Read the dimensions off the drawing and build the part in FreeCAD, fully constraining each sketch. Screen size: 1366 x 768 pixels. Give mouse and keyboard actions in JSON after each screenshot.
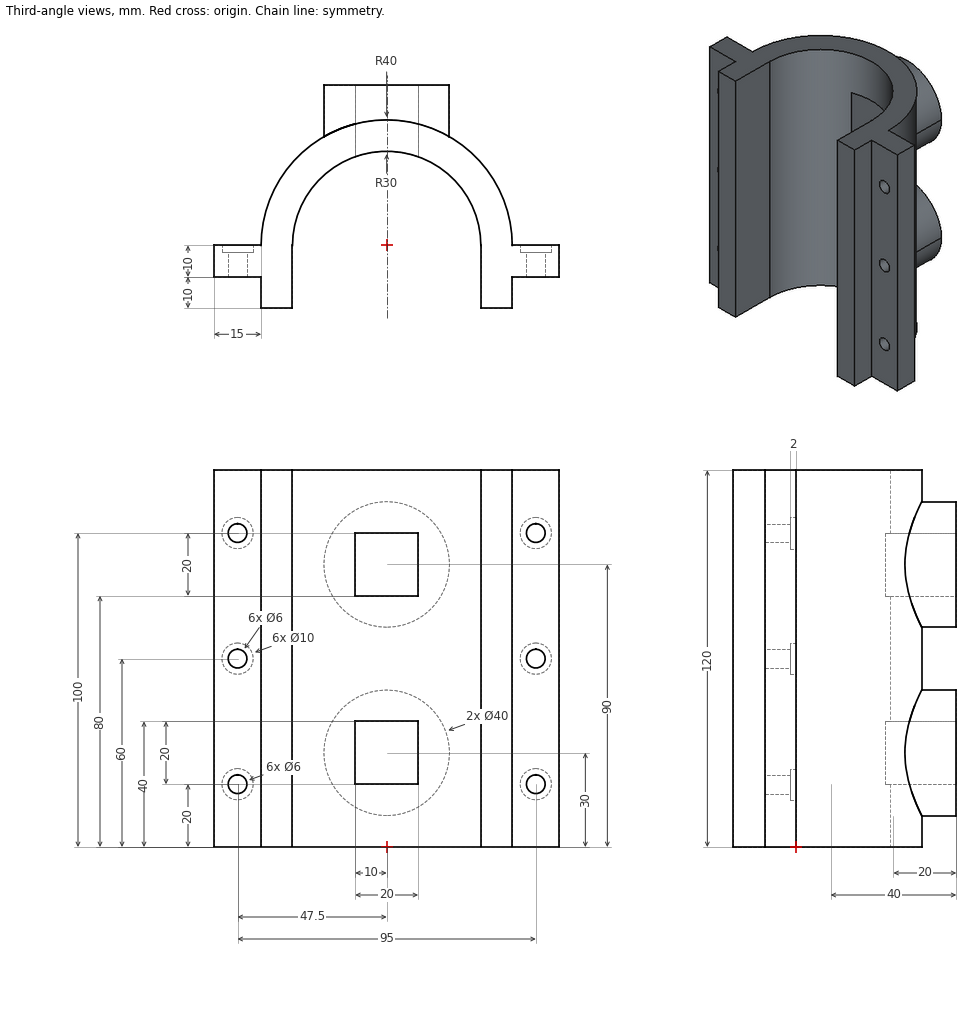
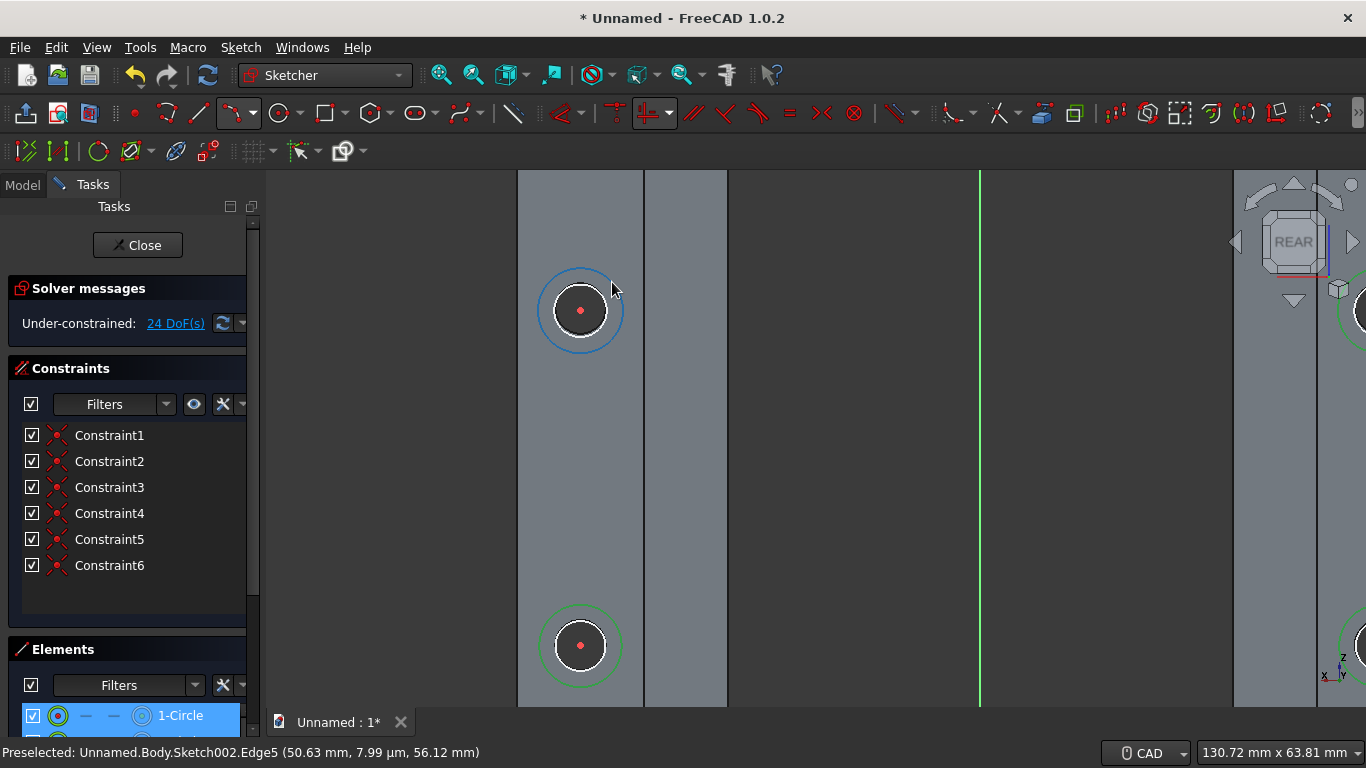
{"action": "left_click", "coordinate": [610, 281]}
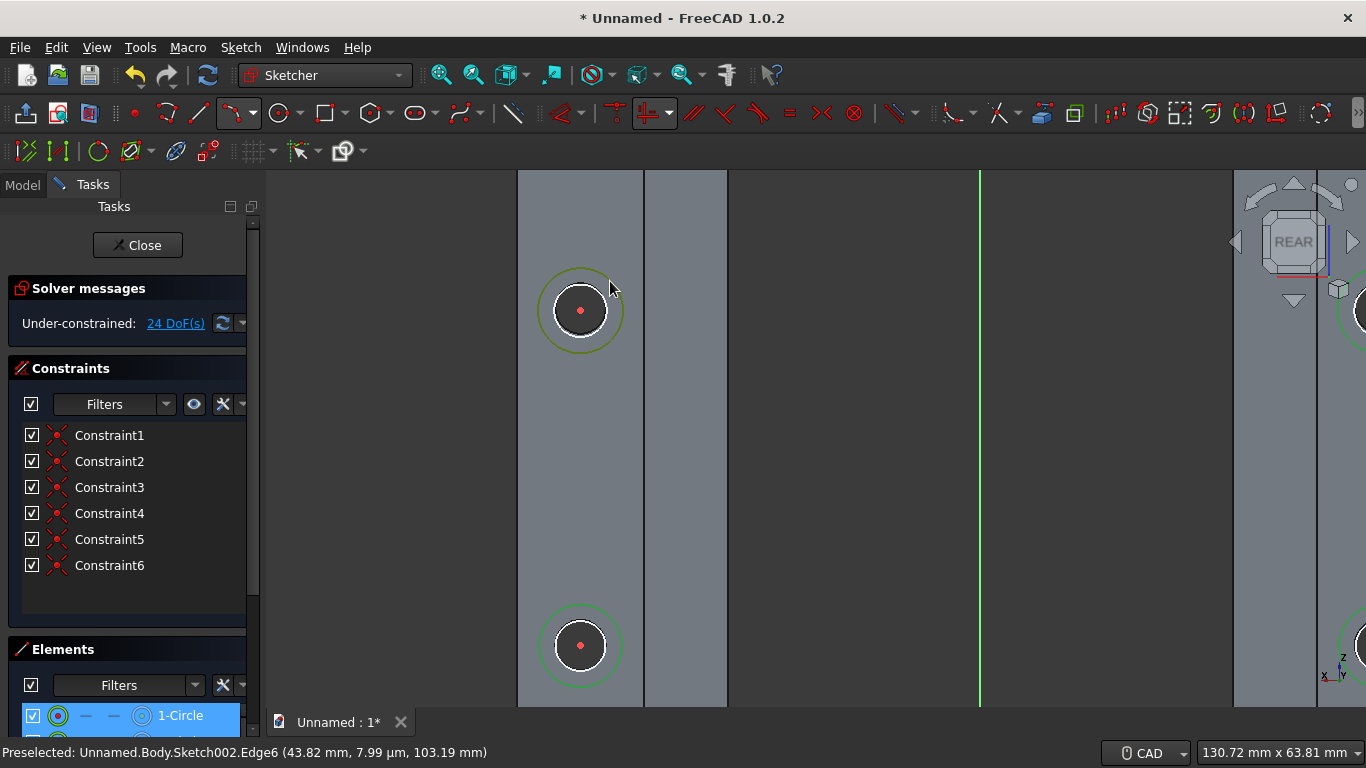
{"action": "left_click", "coordinate": [790, 114]}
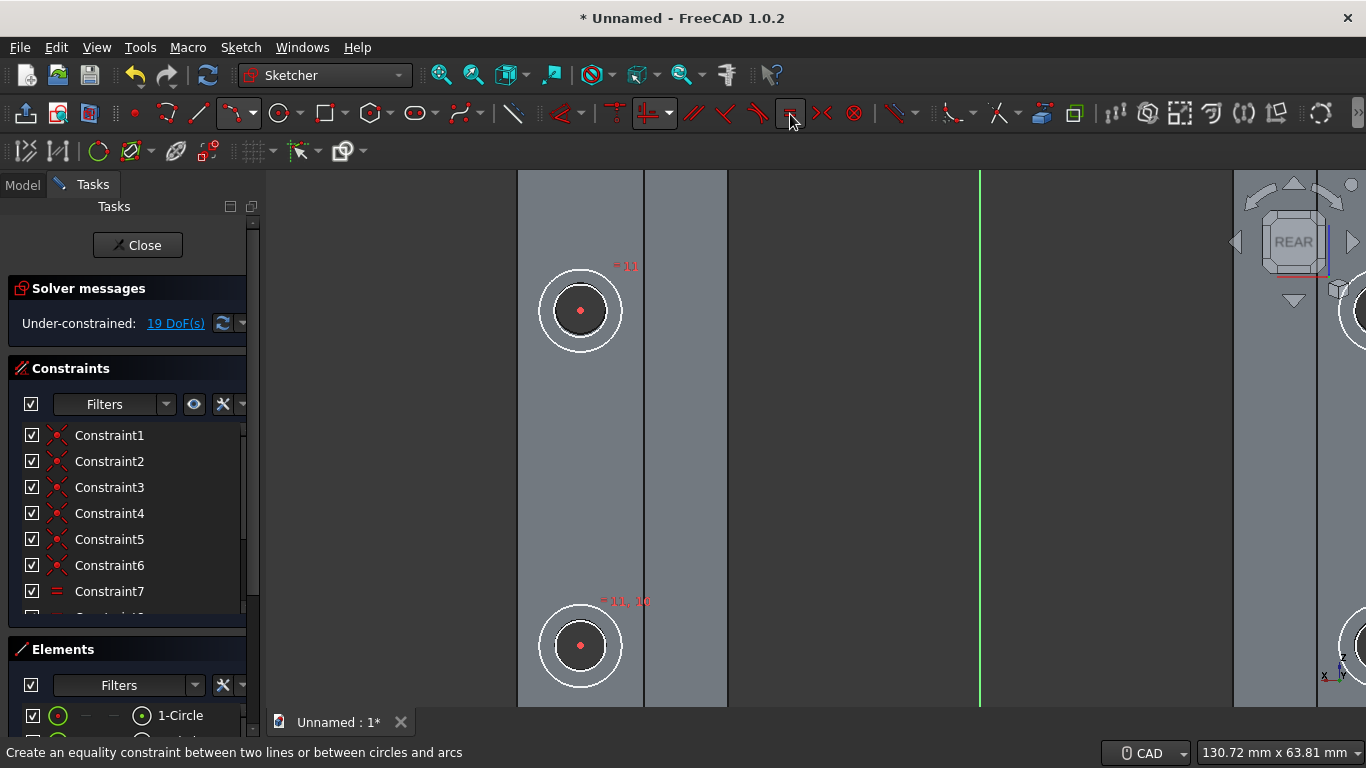
{"action": "scroll", "coordinate": [612, 282], "scroll_direction": "down", "scroll_amount": 5}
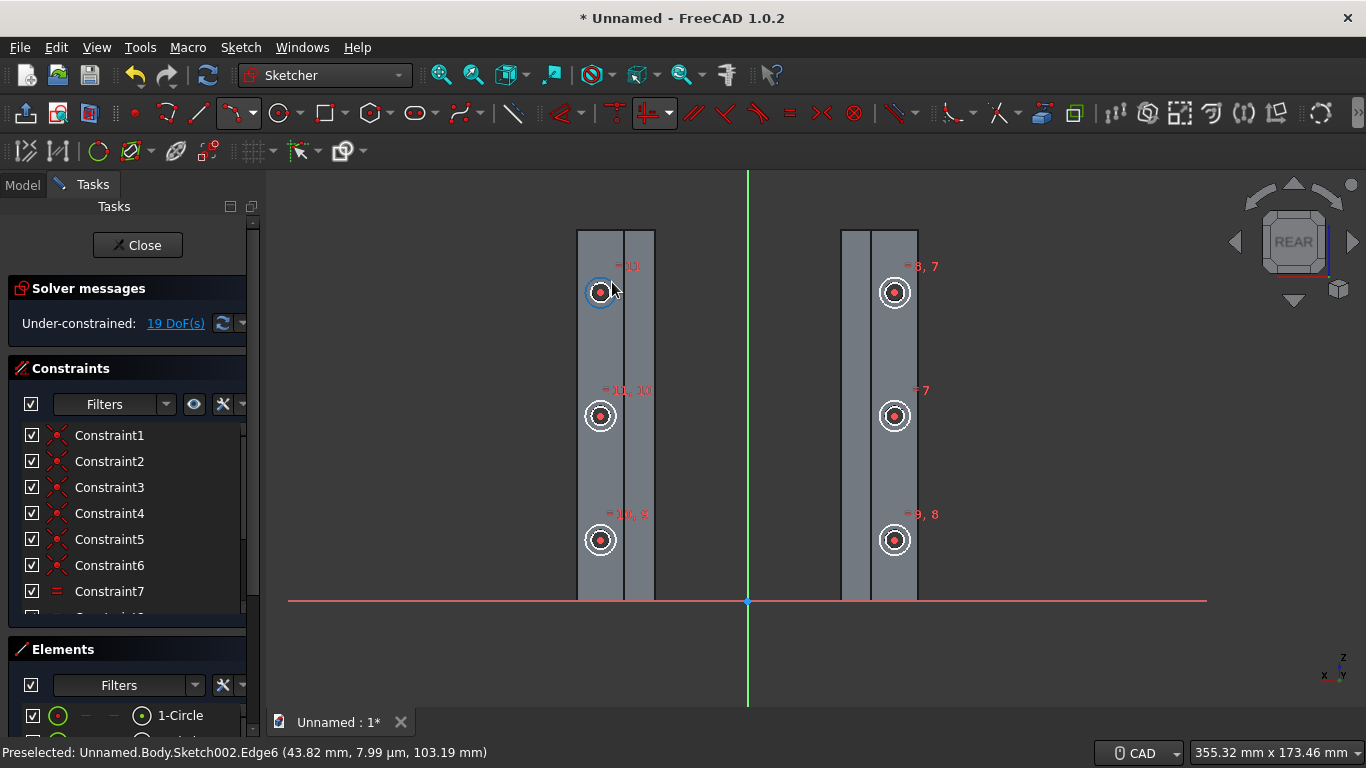
{"action": "scroll", "coordinate": [901, 410], "scroll_direction": "up", "scroll_amount": 5}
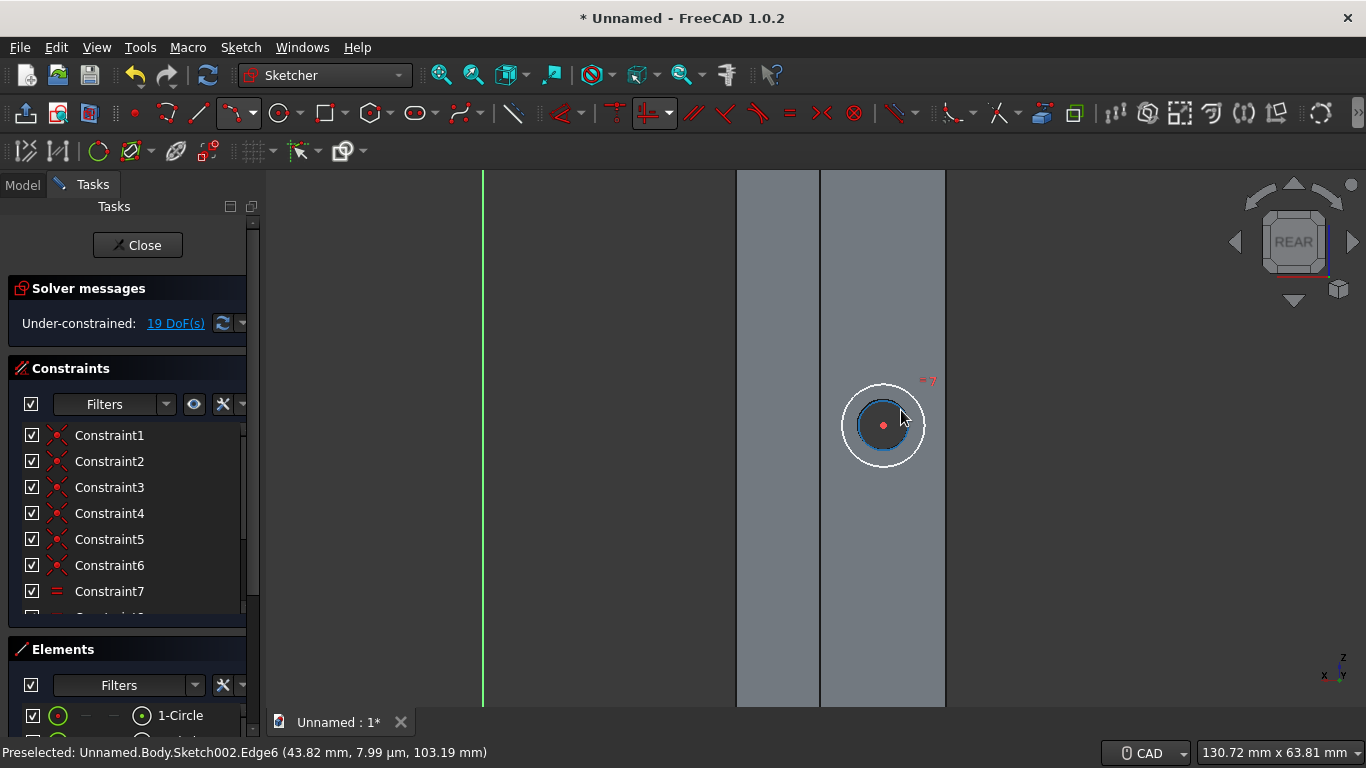
{"action": "left_click", "coordinate": [901, 408]}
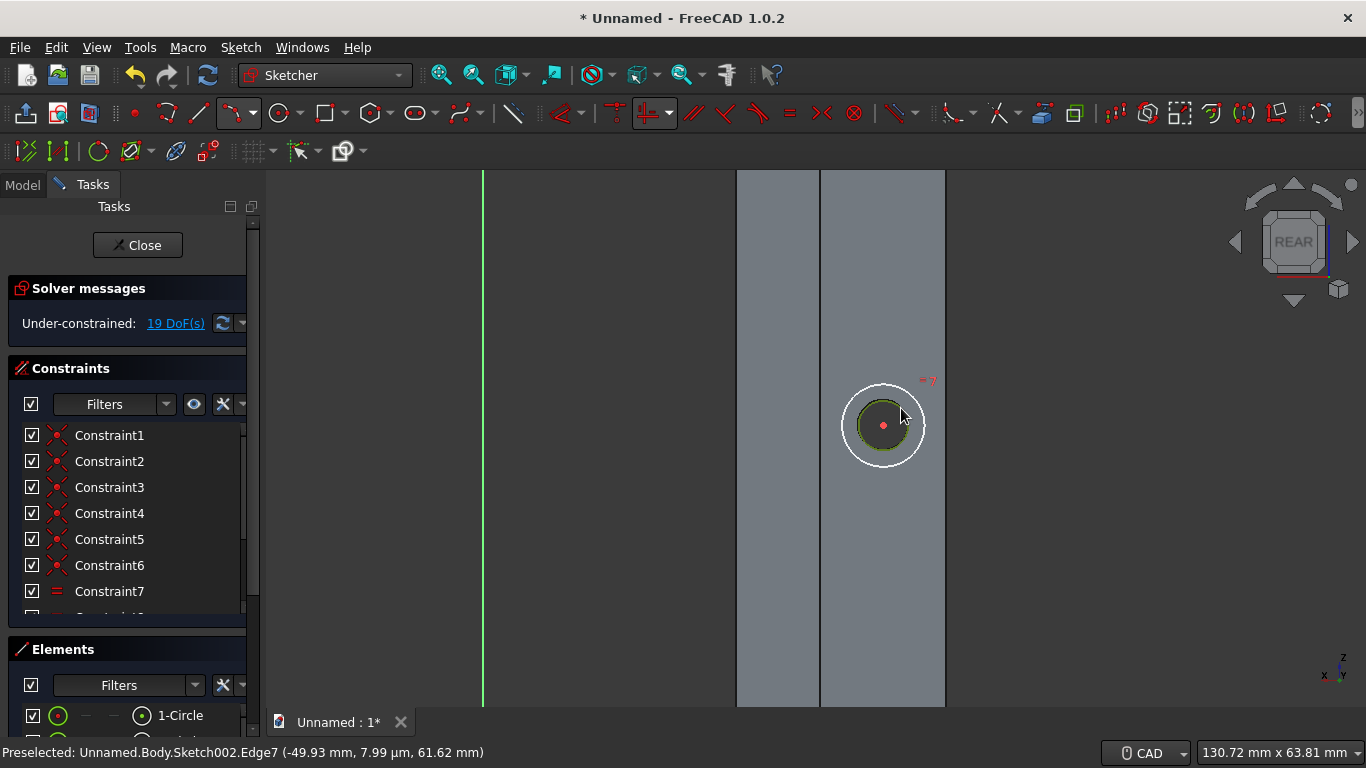
{"action": "scroll", "coordinate": [901, 410], "scroll_direction": "down", "scroll_amount": 5}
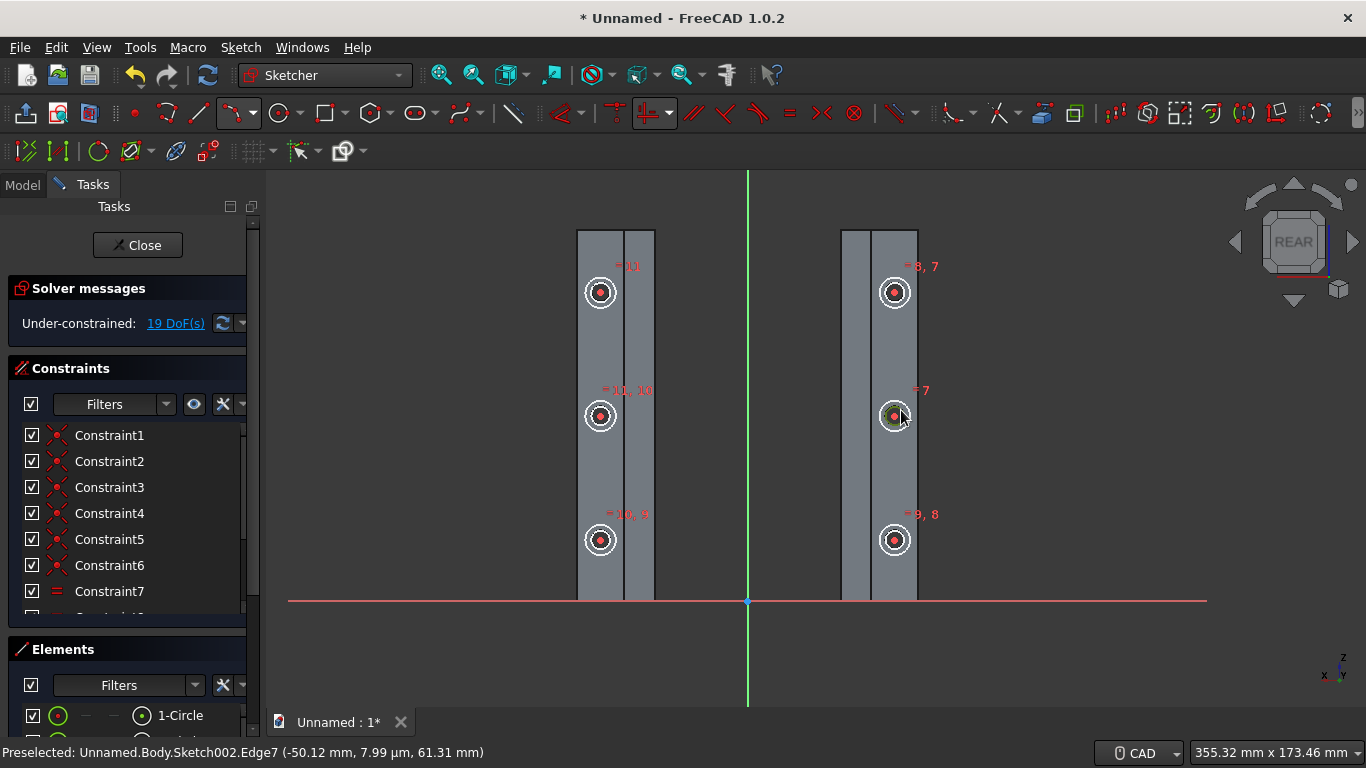
{"action": "scroll", "coordinate": [902, 286], "scroll_direction": "up", "scroll_amount": 5}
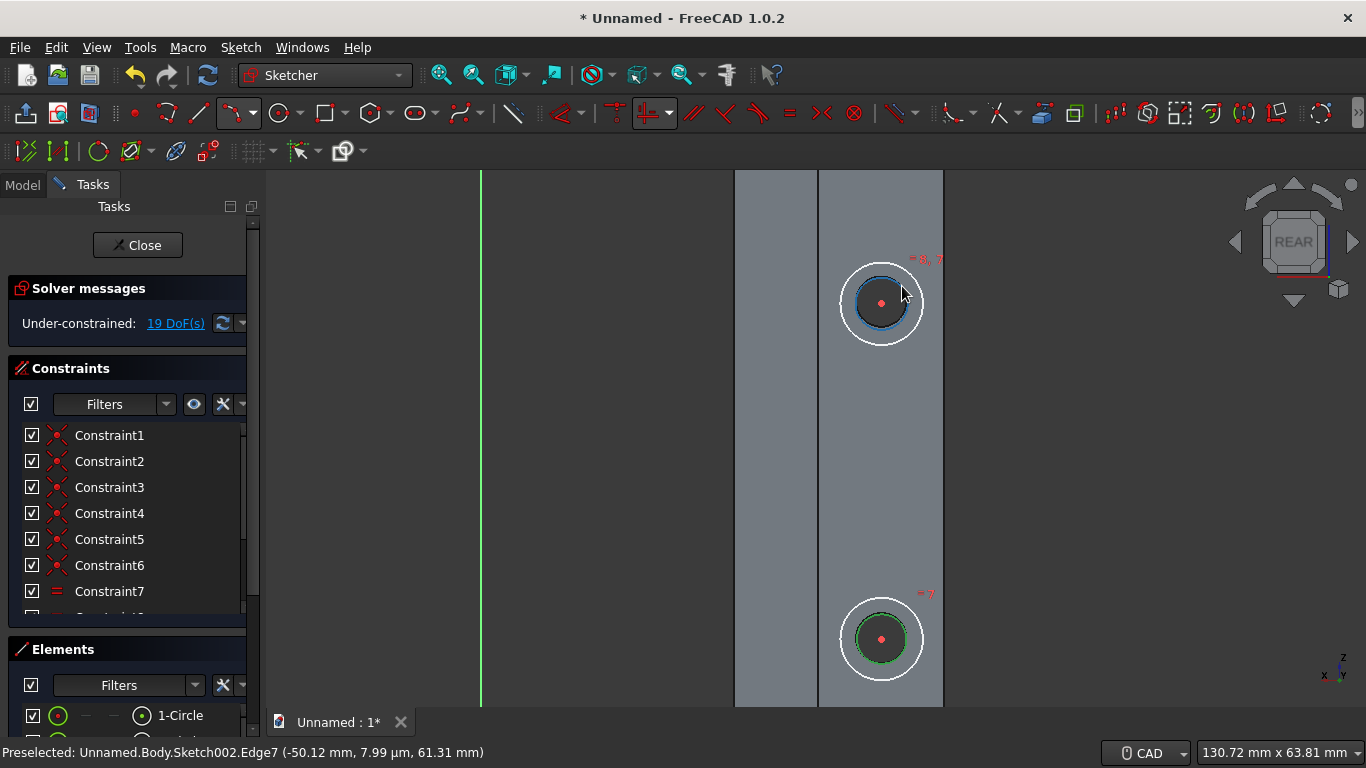
{"action": "left_click", "coordinate": [900, 285]}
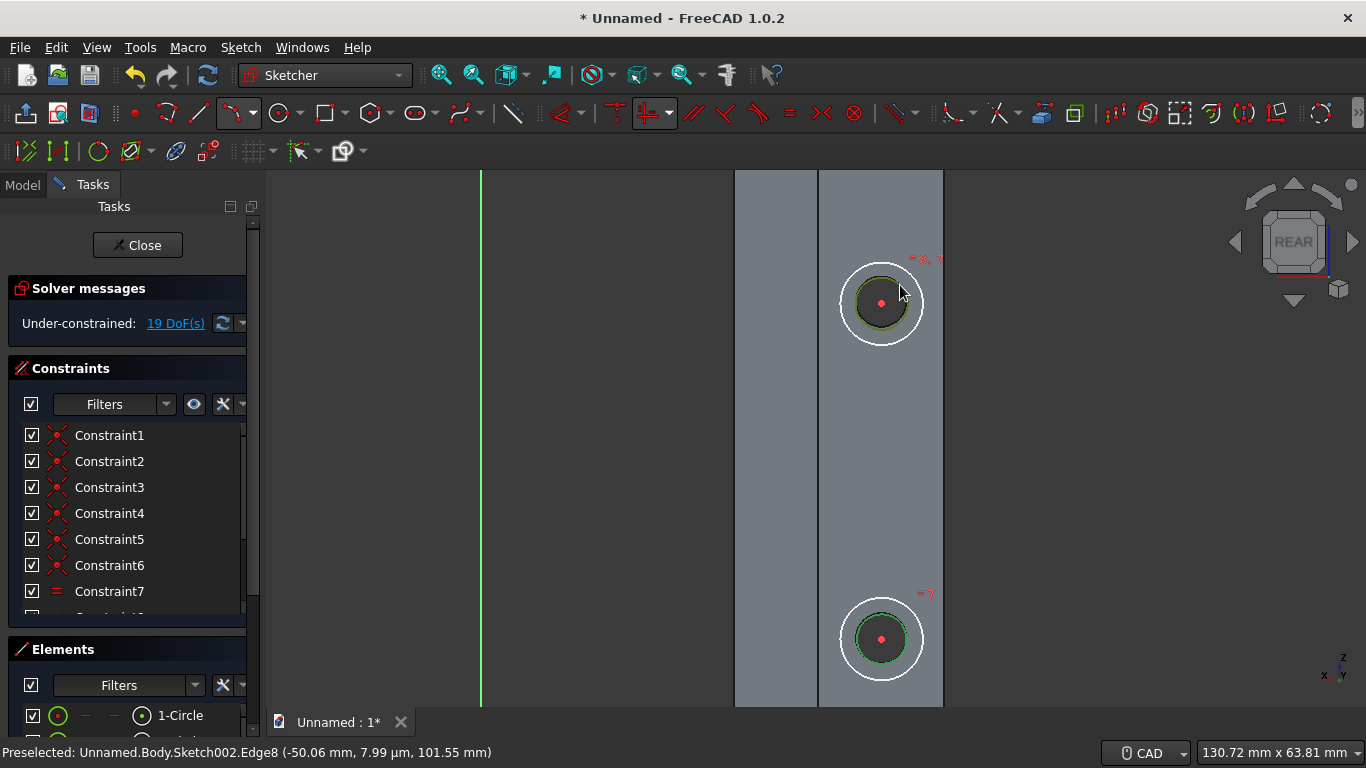
{"action": "scroll", "coordinate": [902, 286], "scroll_direction": "down", "scroll_amount": 5}